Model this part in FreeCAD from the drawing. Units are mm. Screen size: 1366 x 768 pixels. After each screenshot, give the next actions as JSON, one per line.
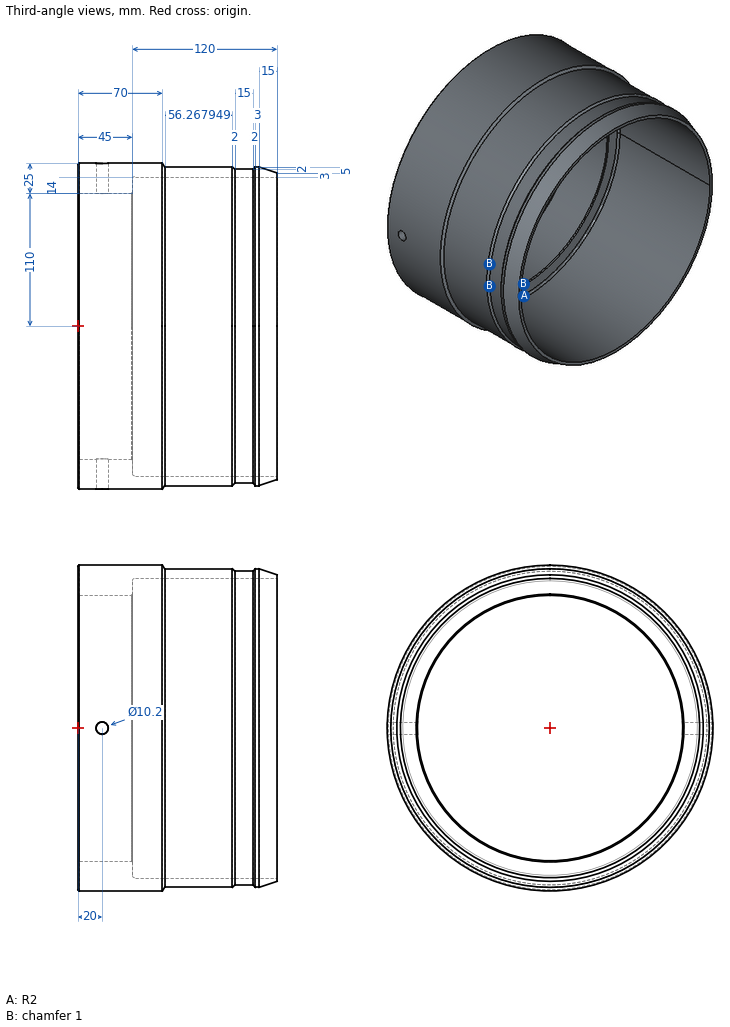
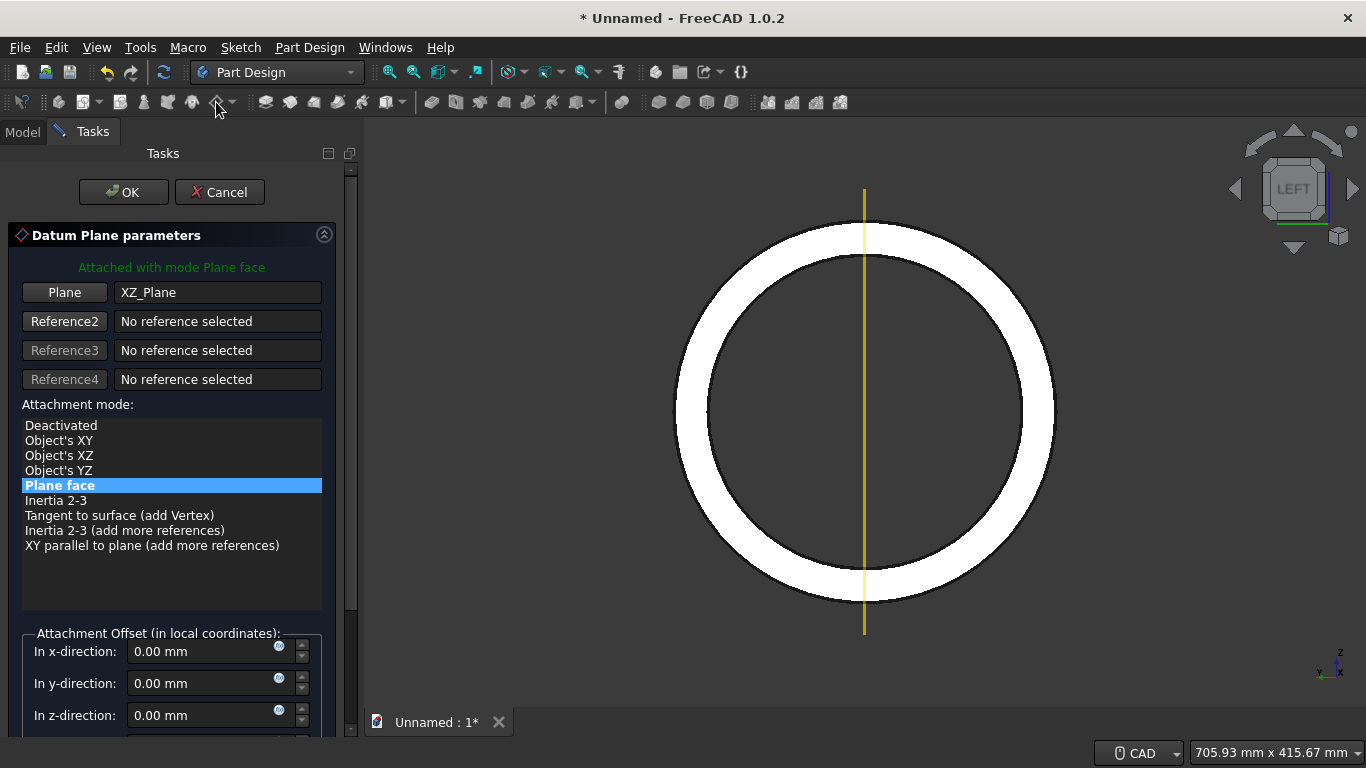
{"action": "triple_click", "coordinate": [210, 715]}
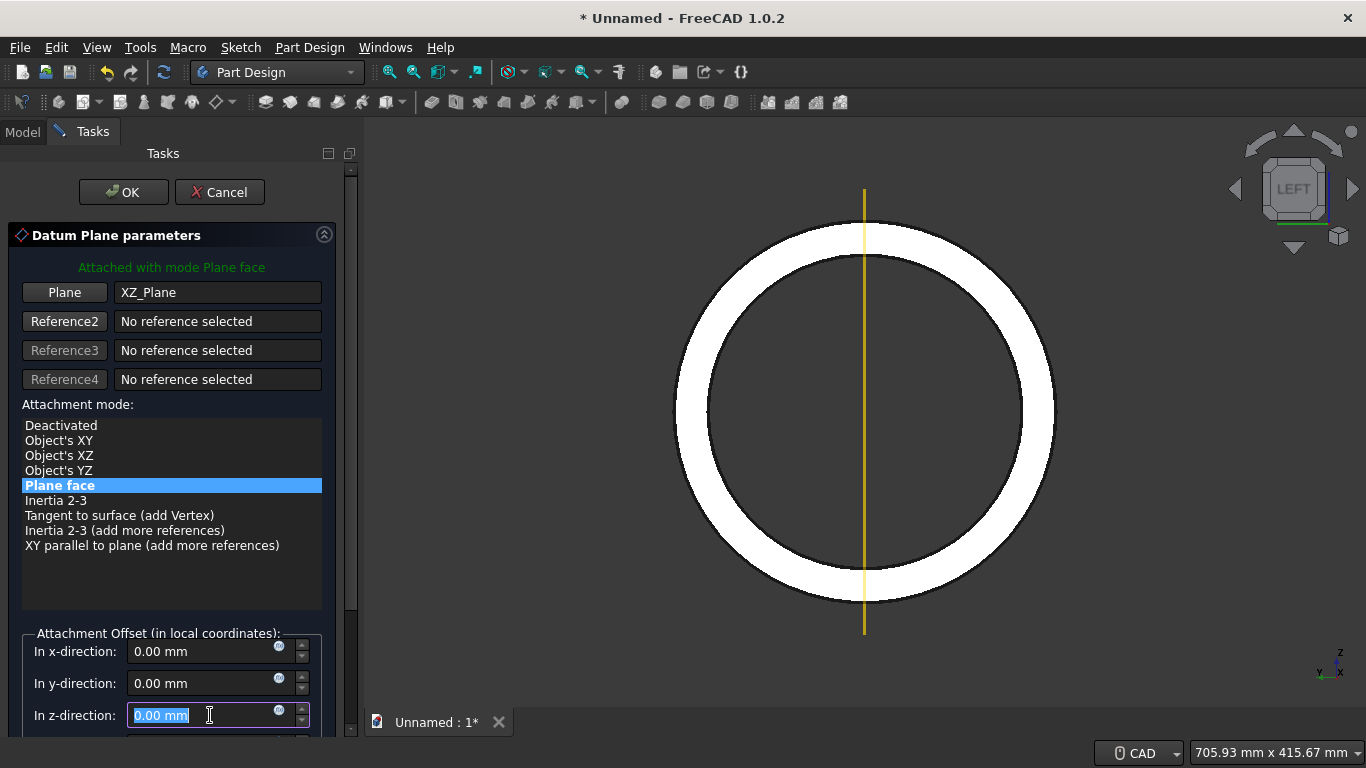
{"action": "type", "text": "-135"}
{"action": "key", "text": "Tab"}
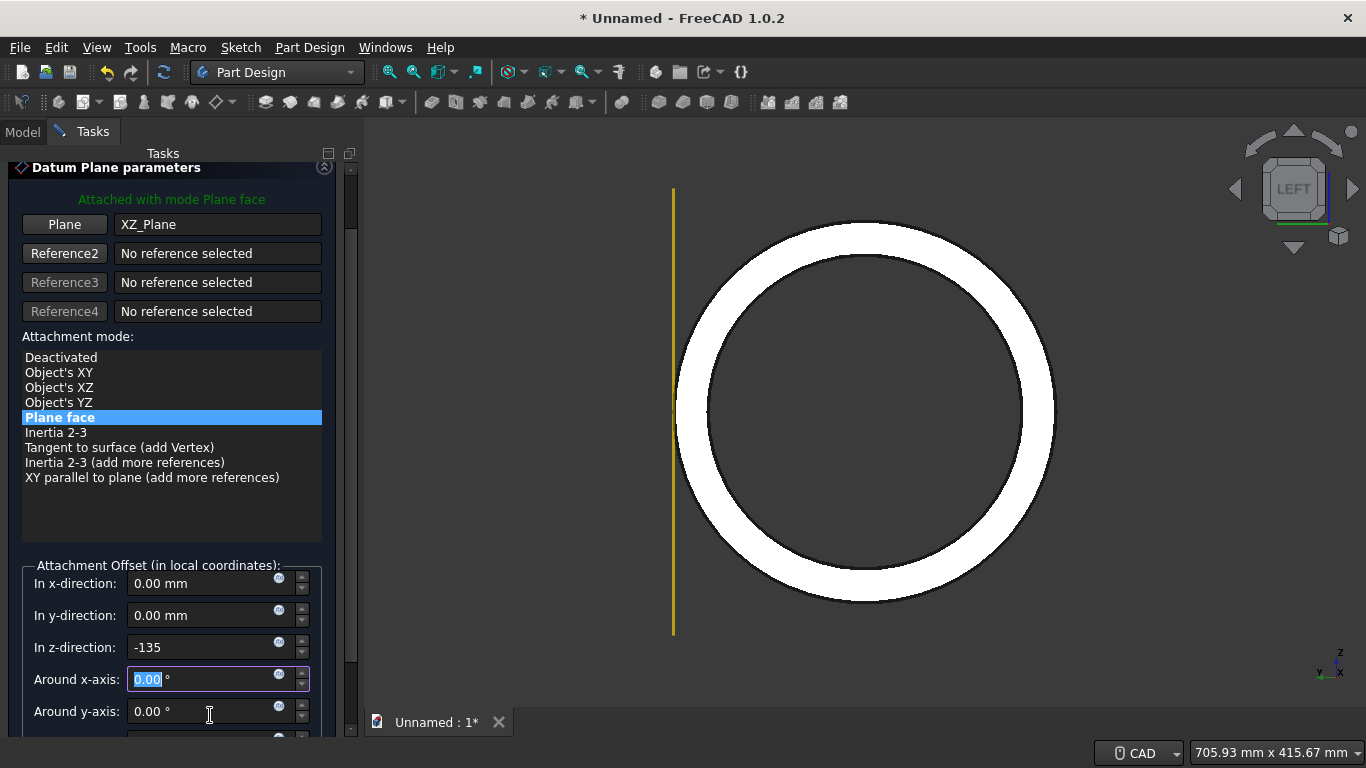
{"action": "scroll", "coordinate": [351, 450], "scroll_direction": "up", "scroll_amount": 2}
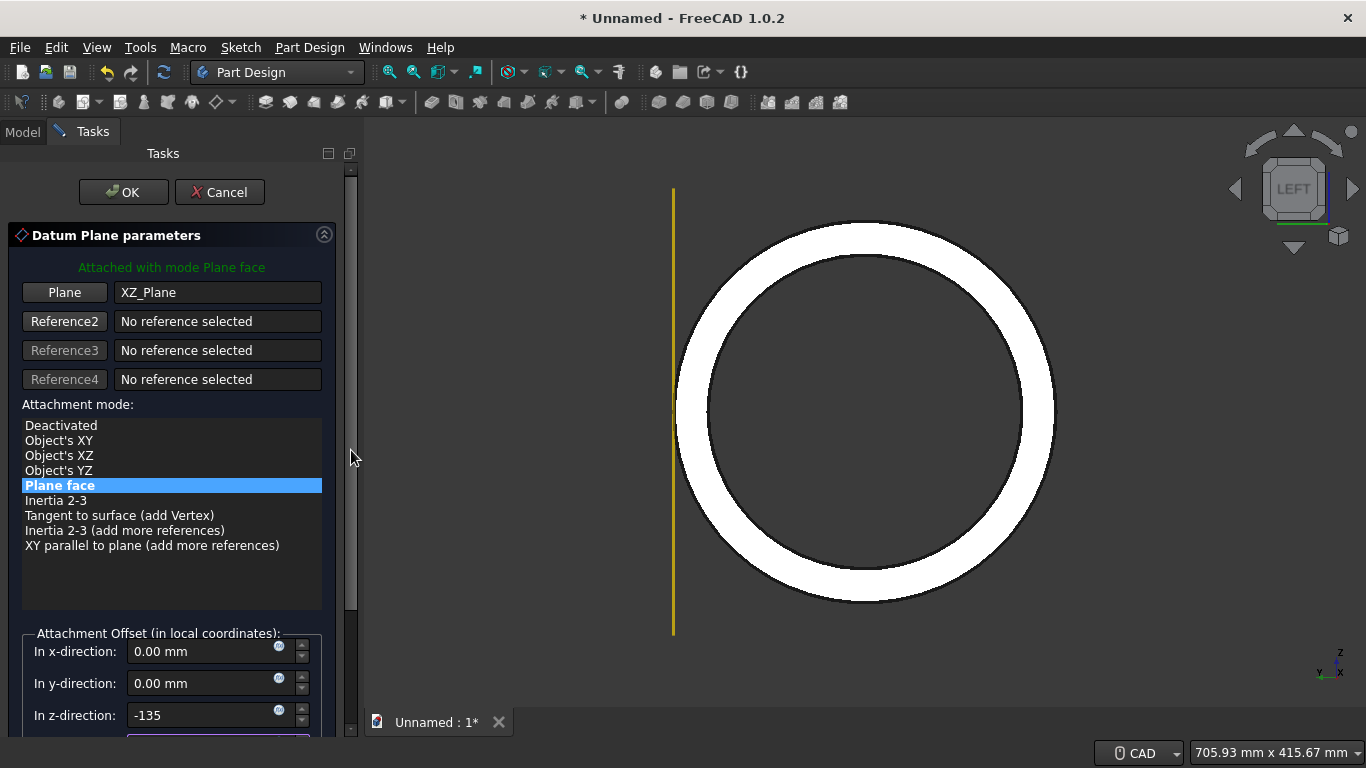
{"action": "left_click", "coordinate": [124, 192]}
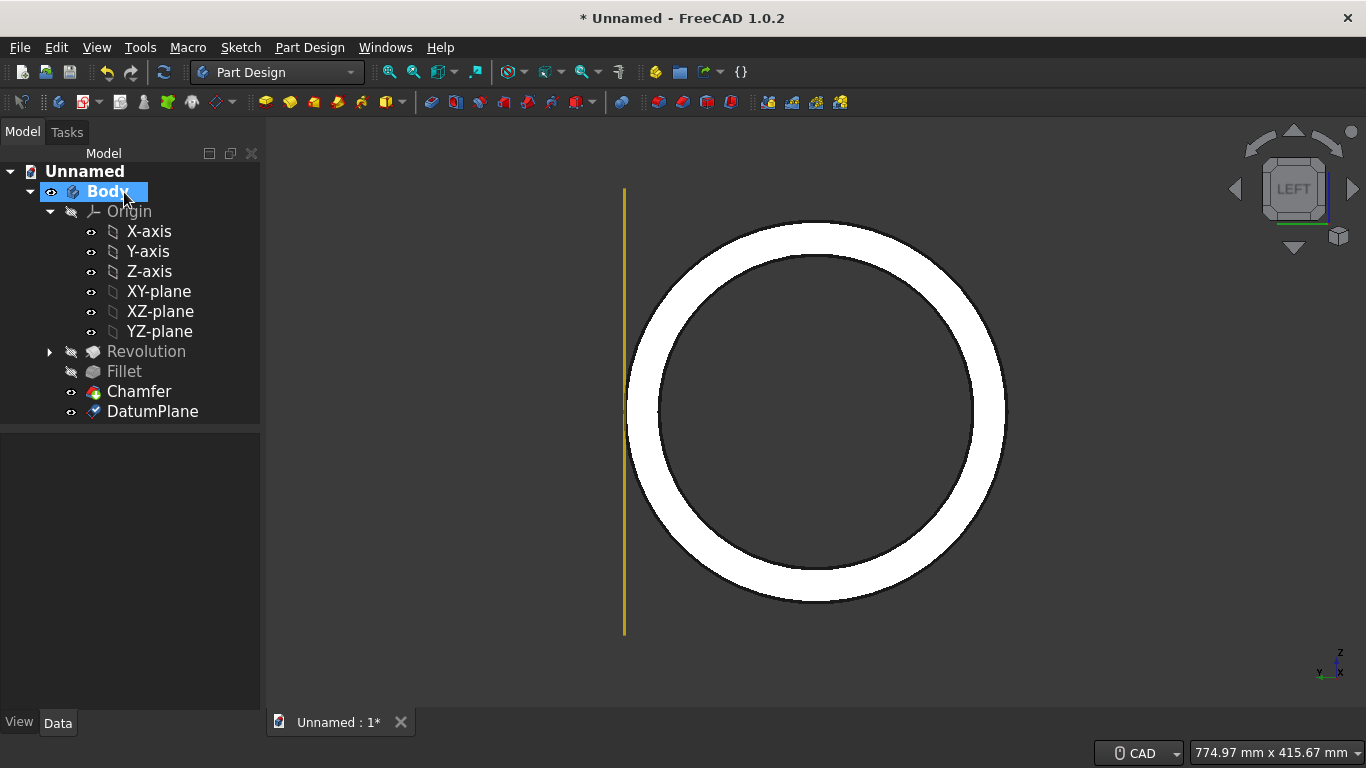
{"action": "left_click", "coordinate": [116, 412]}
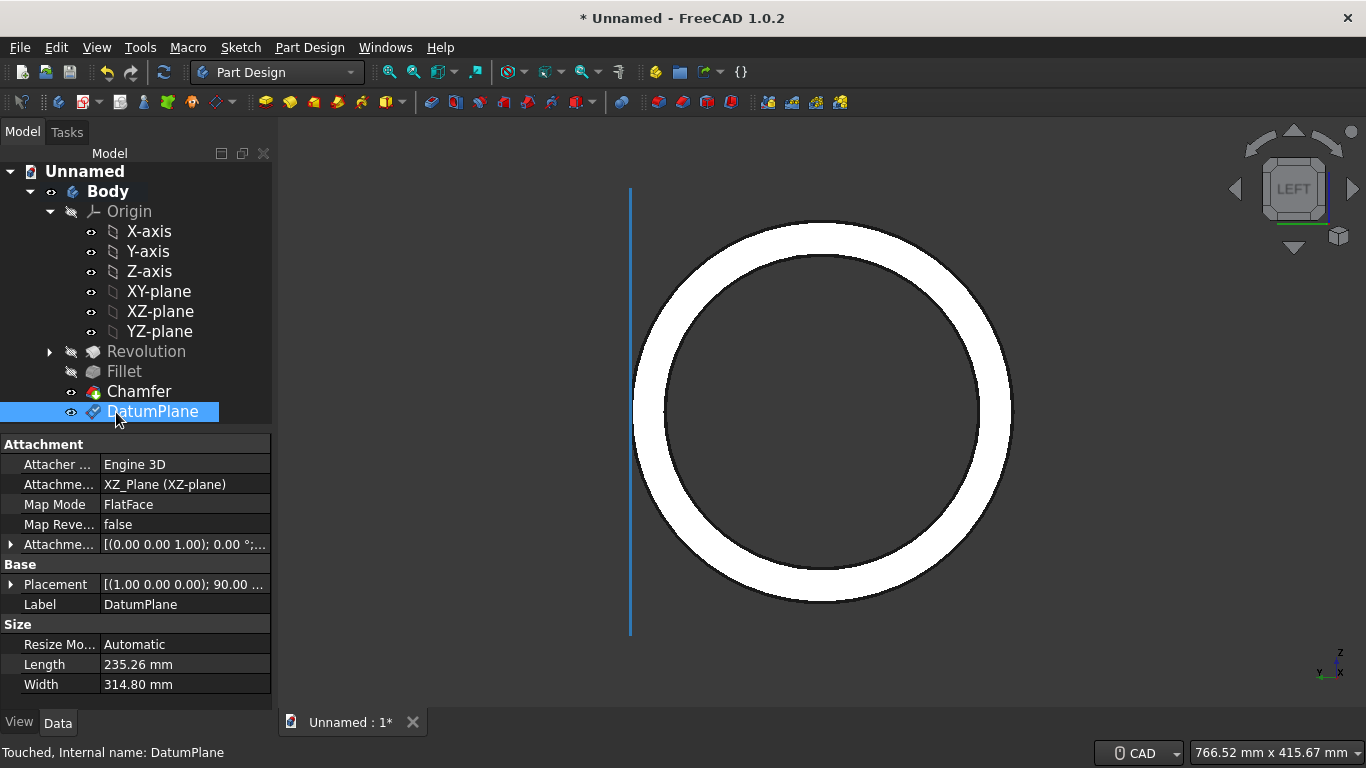
{"action": "left_click", "coordinate": [84, 102]}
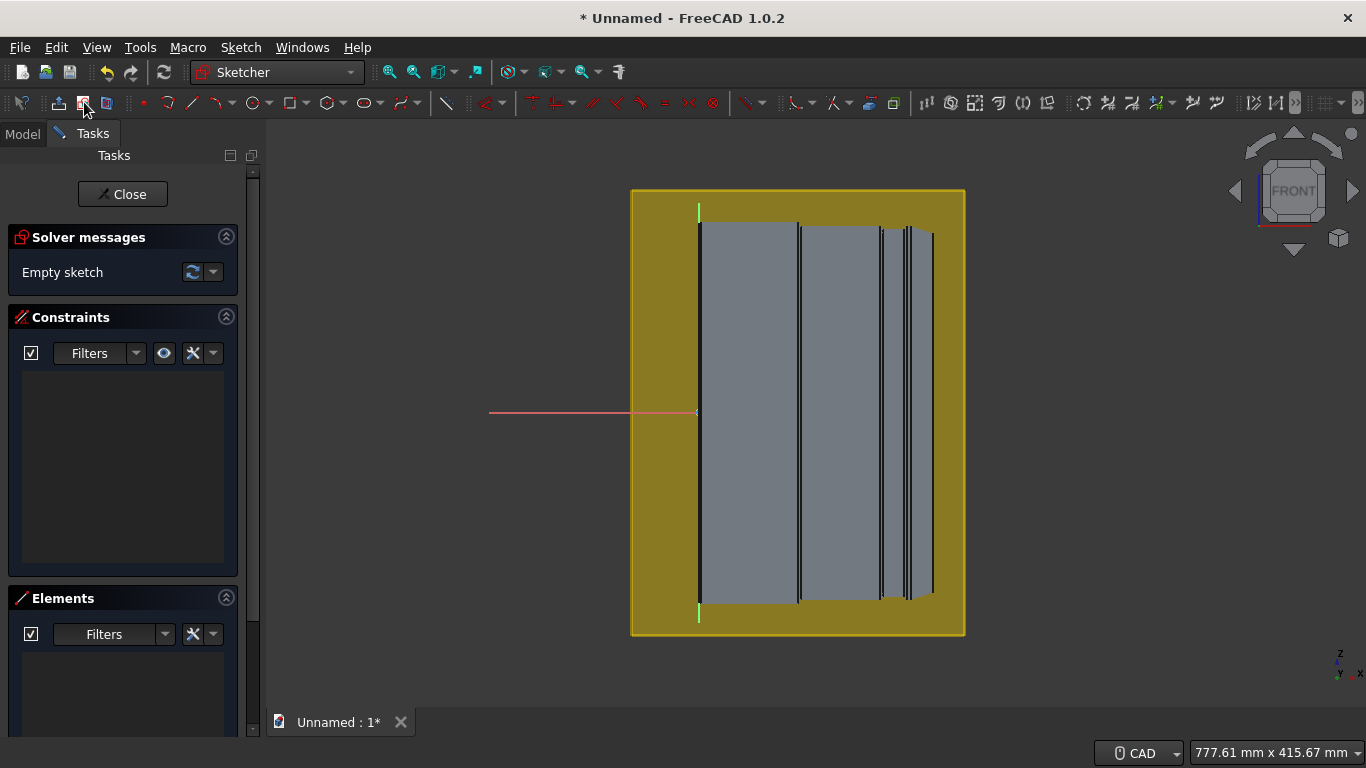
{"action": "left_click", "coordinate": [108, 104]}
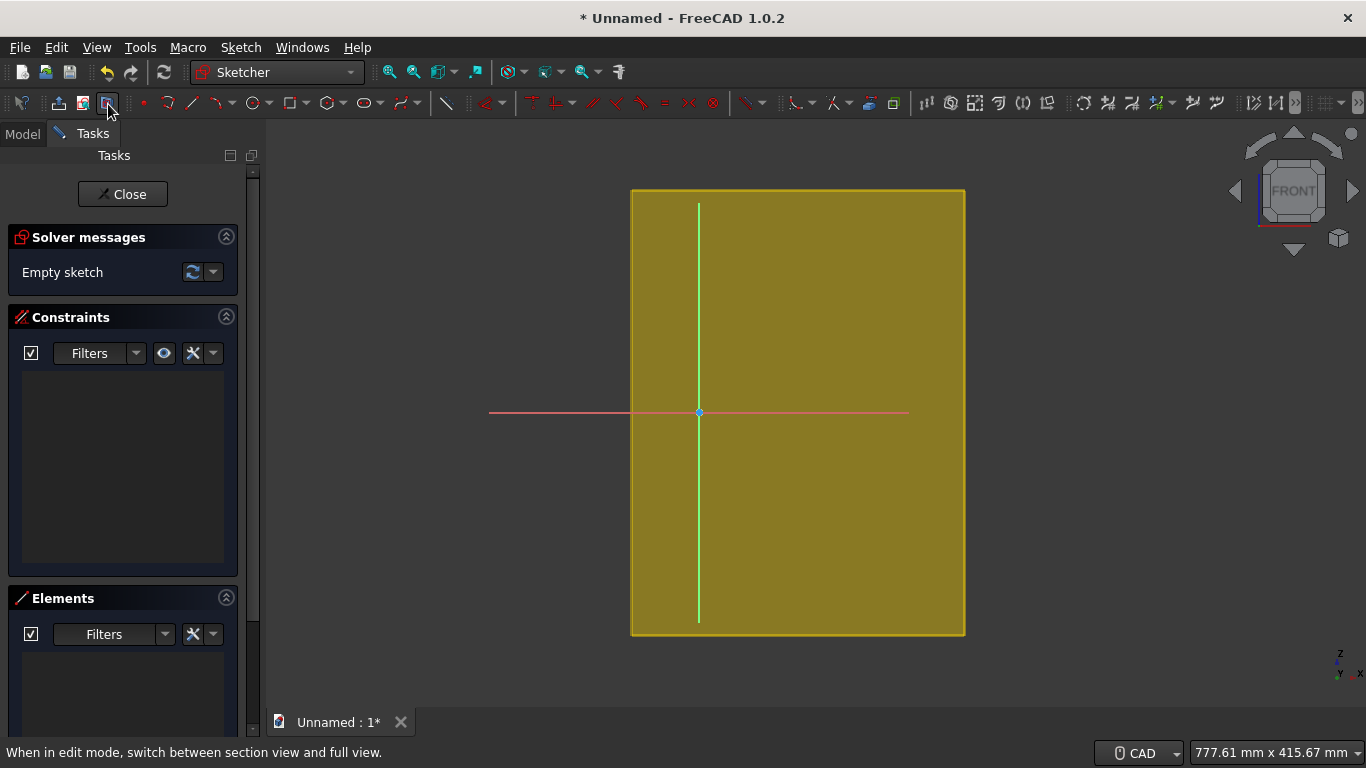
{"action": "scroll", "coordinate": [715, 413], "scroll_direction": "up", "scroll_amount": 14}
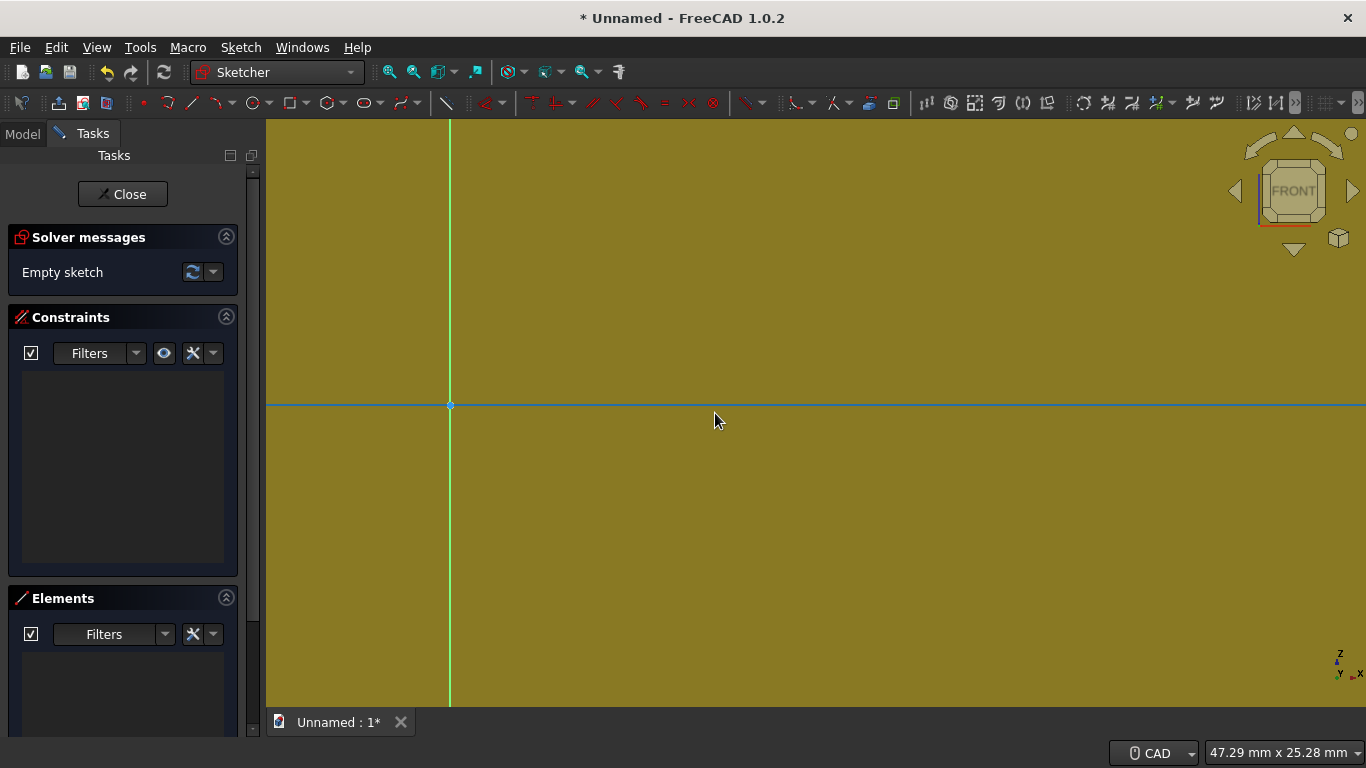
{"action": "left_click", "coordinate": [254, 104]}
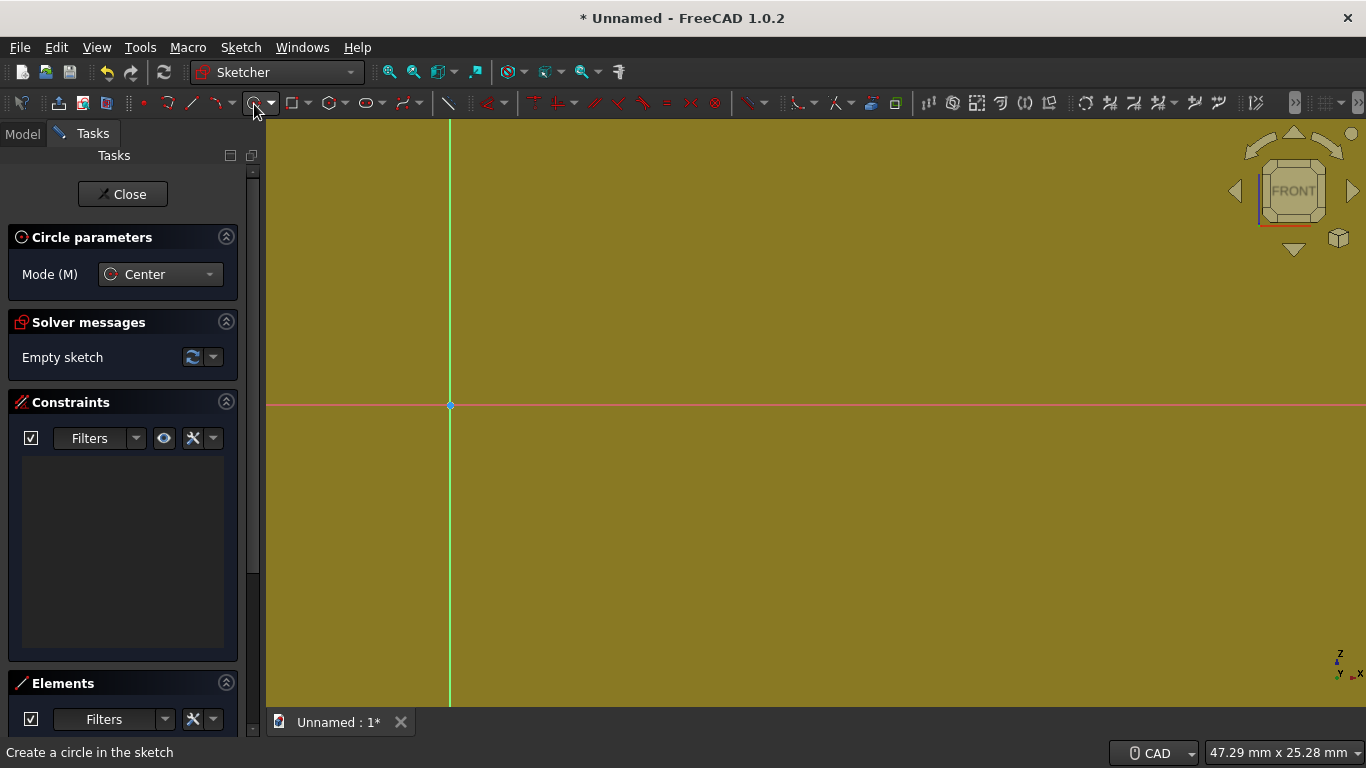
{"action": "left_click", "coordinate": [916, 405]}
{"action": "mouse_move", "coordinate": [1000, 321]}